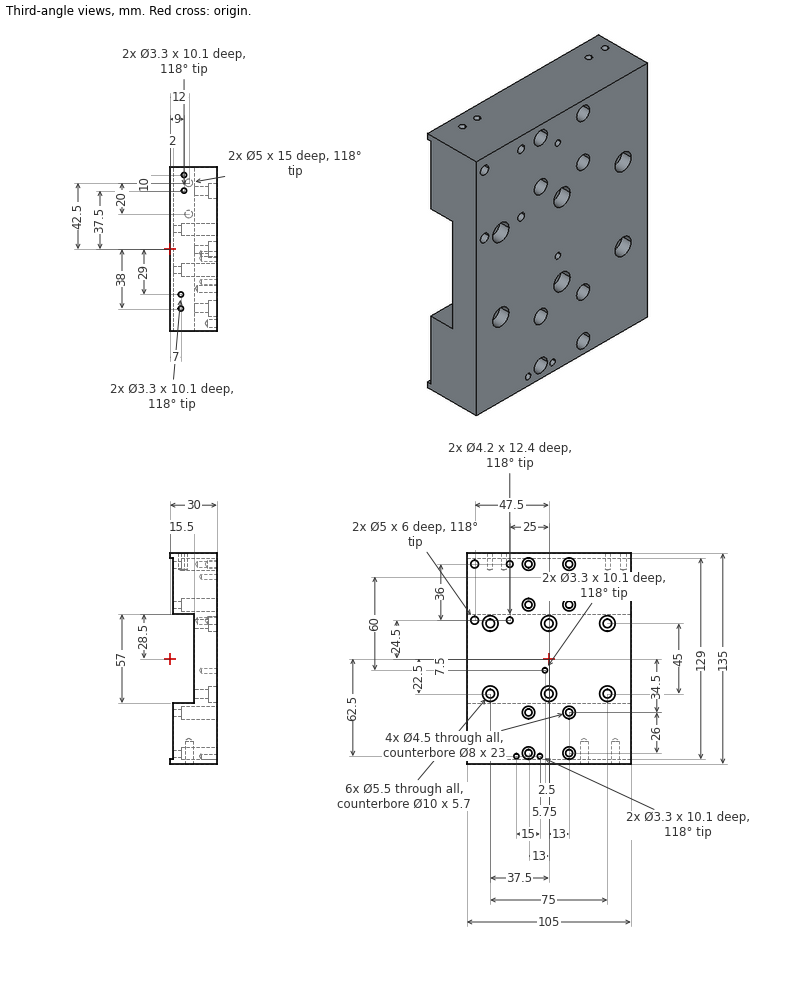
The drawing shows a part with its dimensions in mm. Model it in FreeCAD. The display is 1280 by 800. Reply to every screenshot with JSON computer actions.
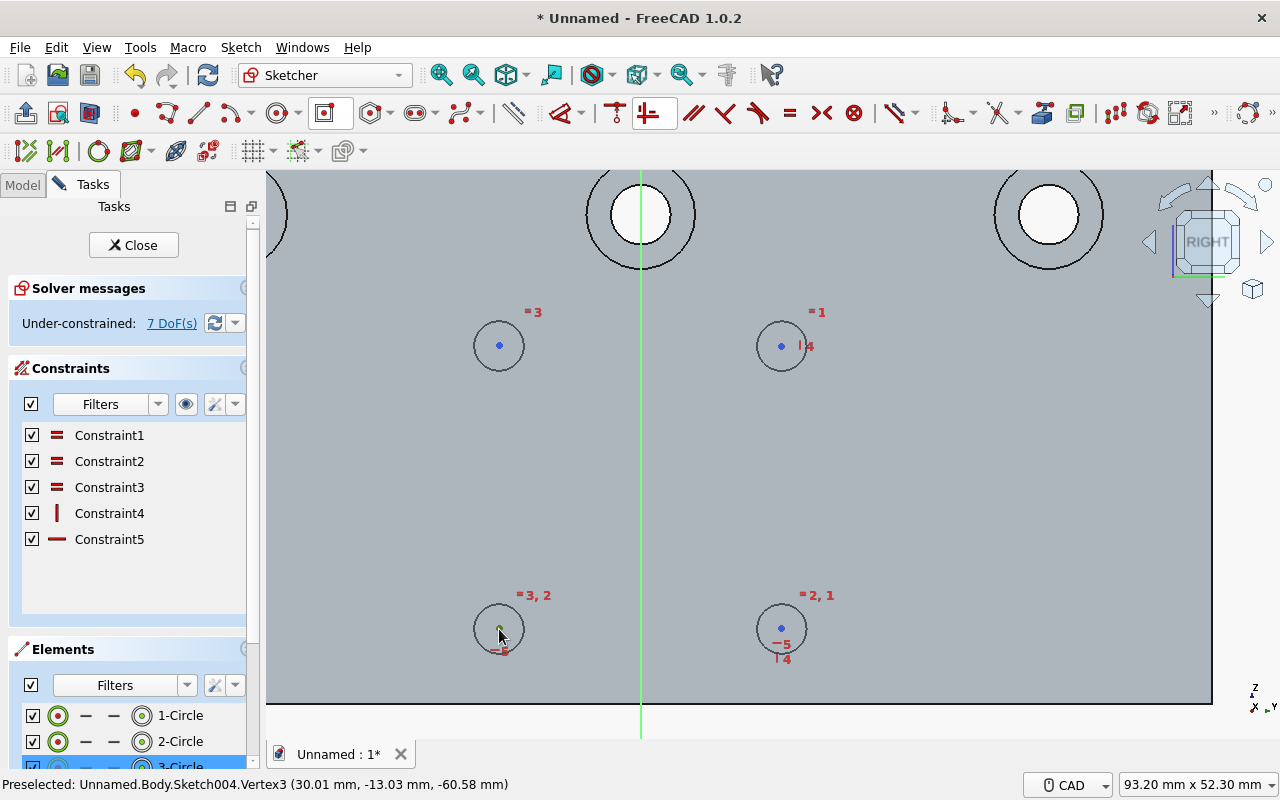
{"action": "left_click", "coordinate": [499, 346]}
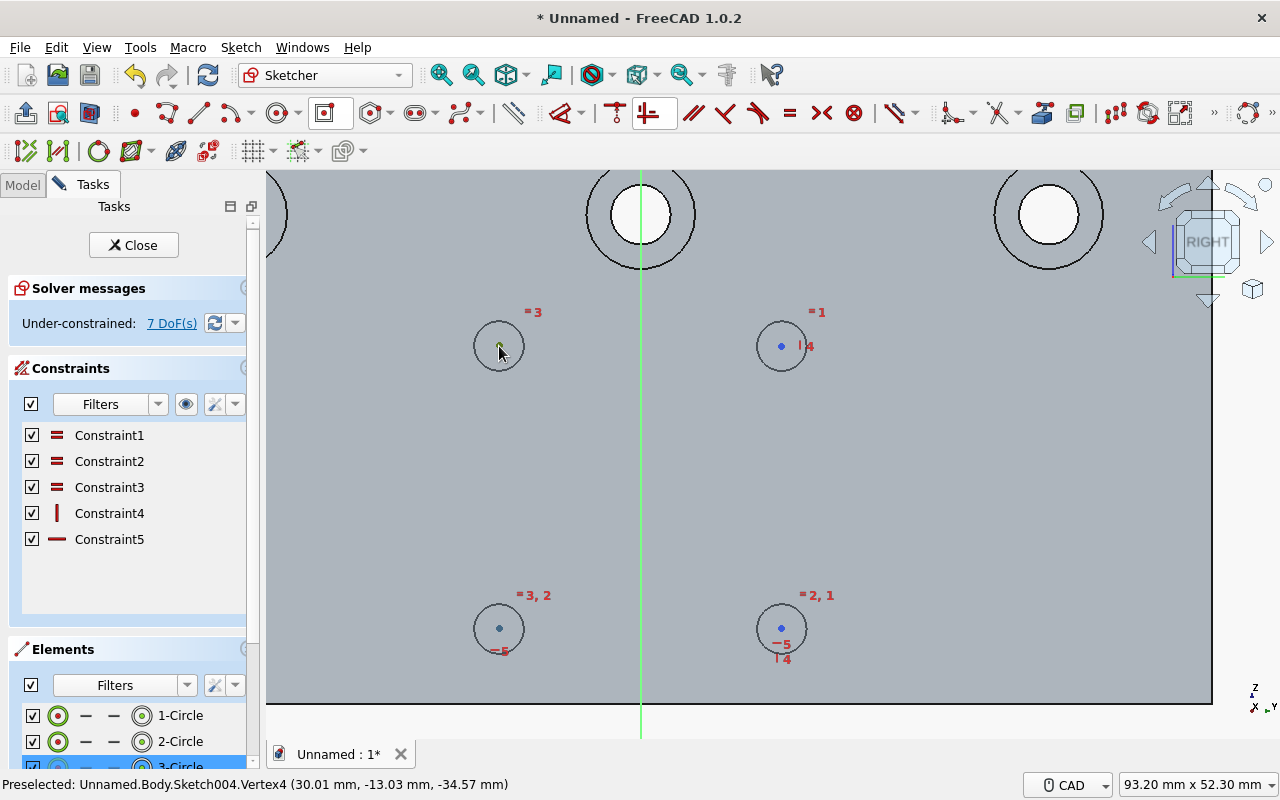
{"action": "key", "text": "v"}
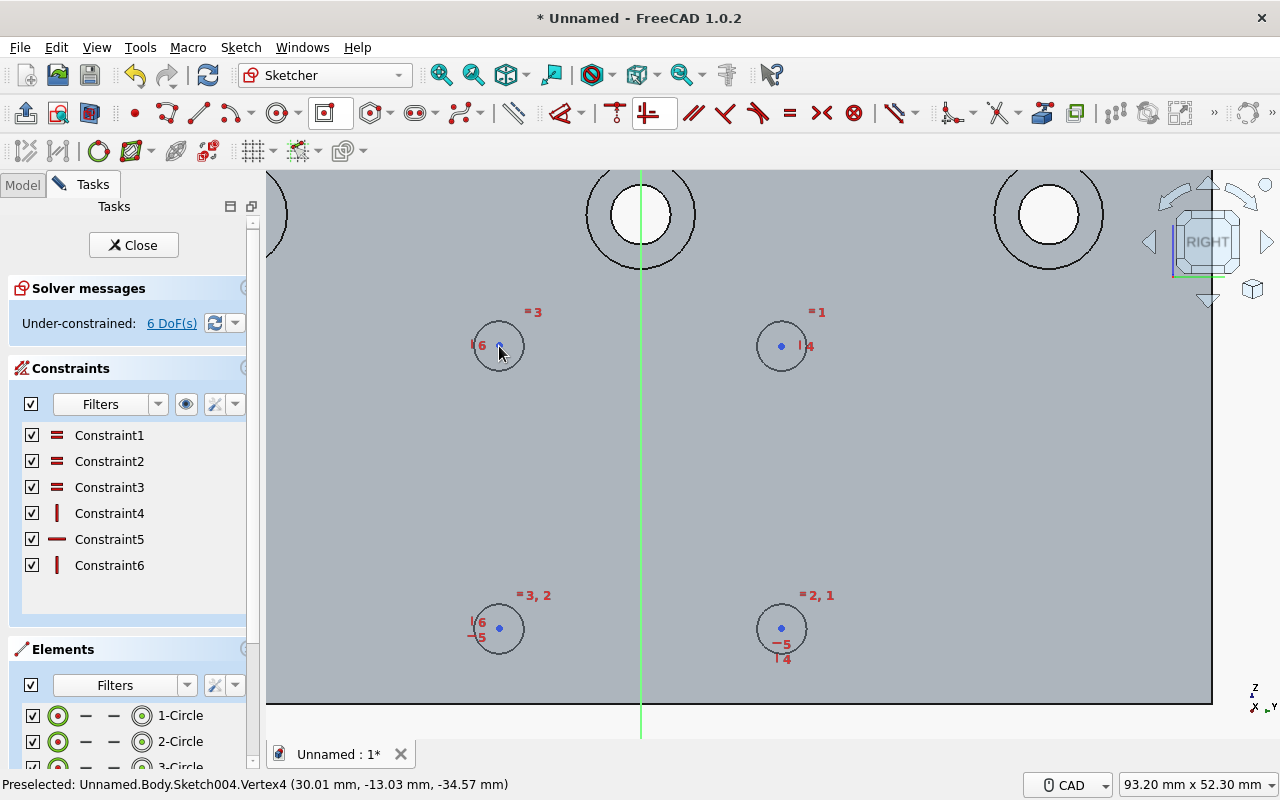
{"action": "left_click", "coordinate": [782, 346]}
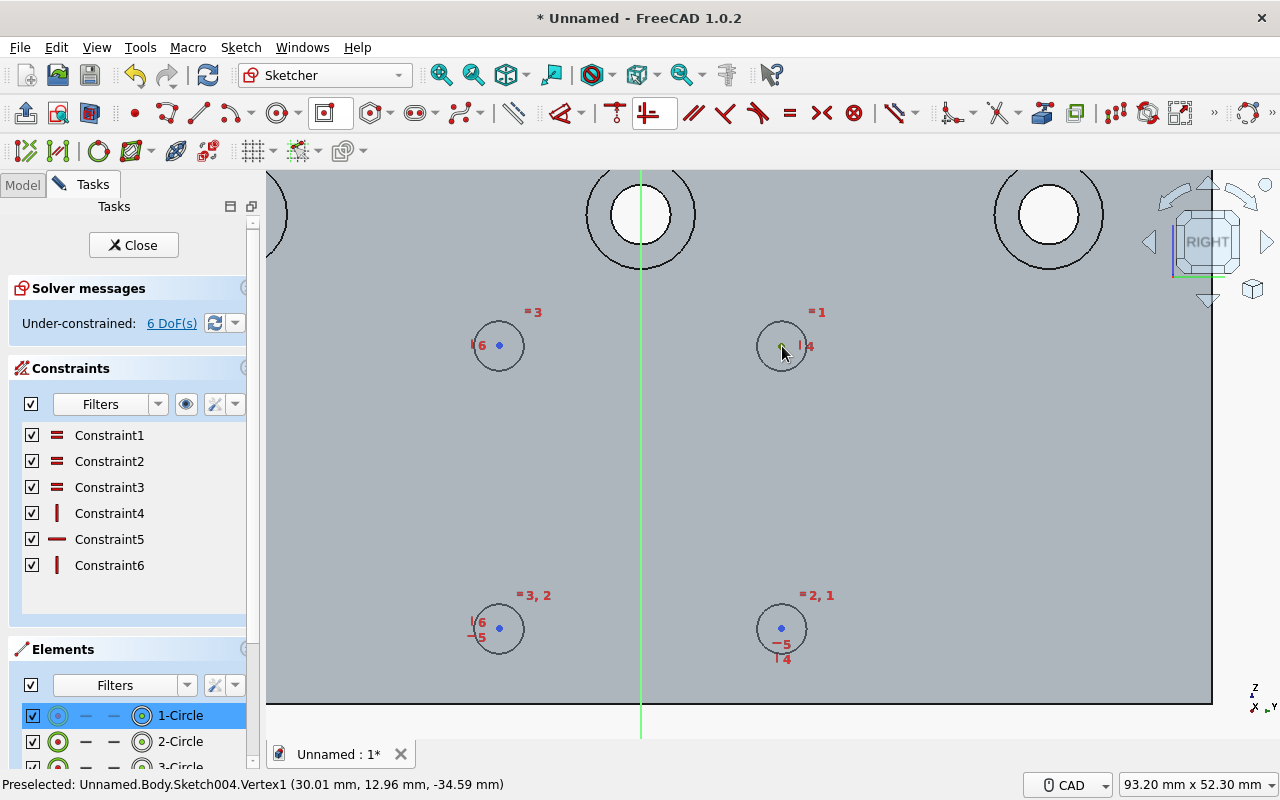
{"action": "left_click", "coordinate": [499, 346]}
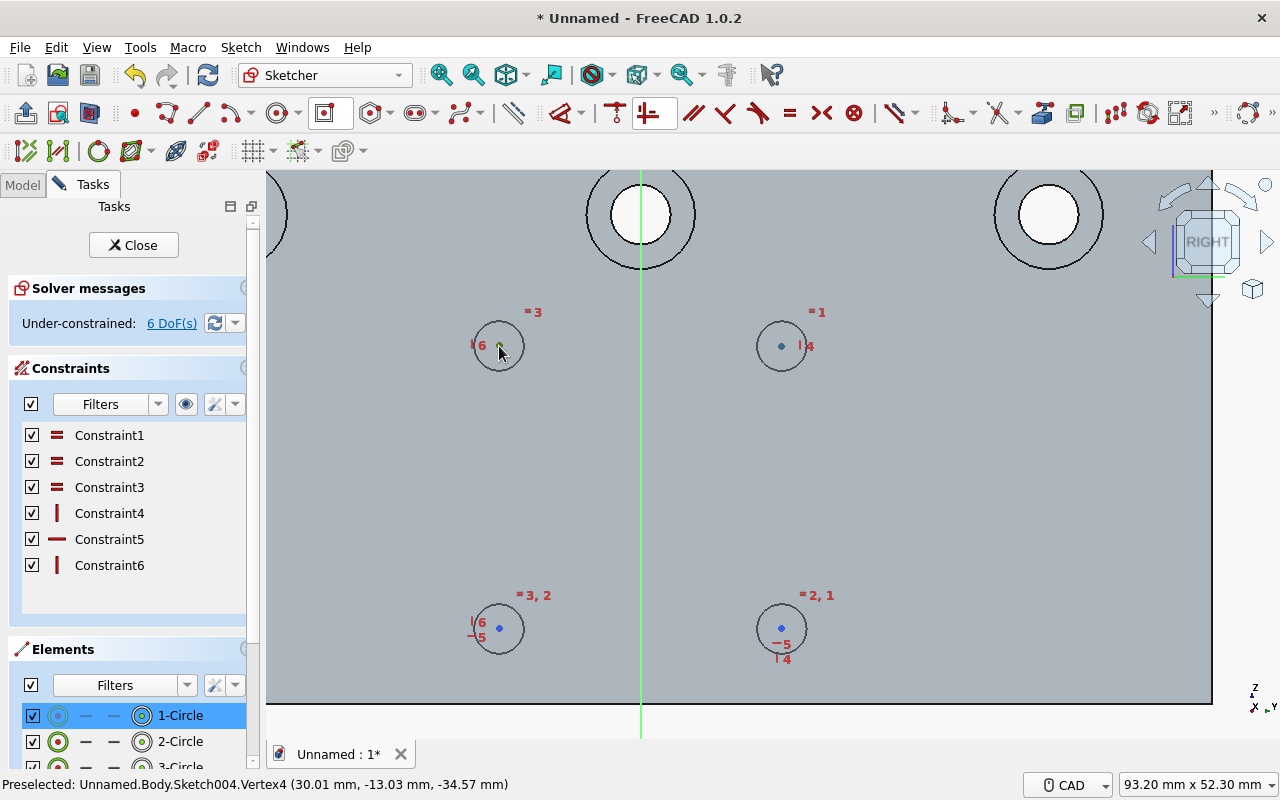
{"action": "left_click", "coordinate": [672, 114]}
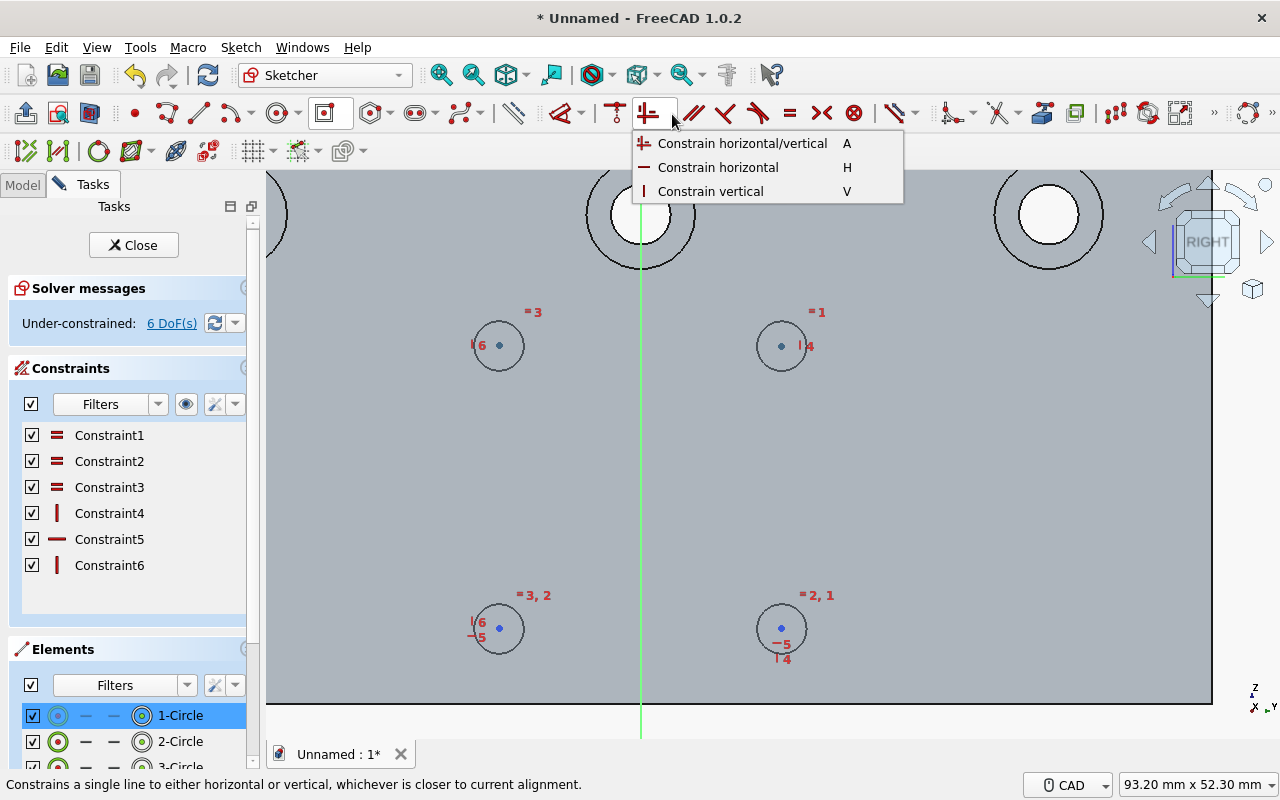
{"action": "left_click", "coordinate": [768, 167]}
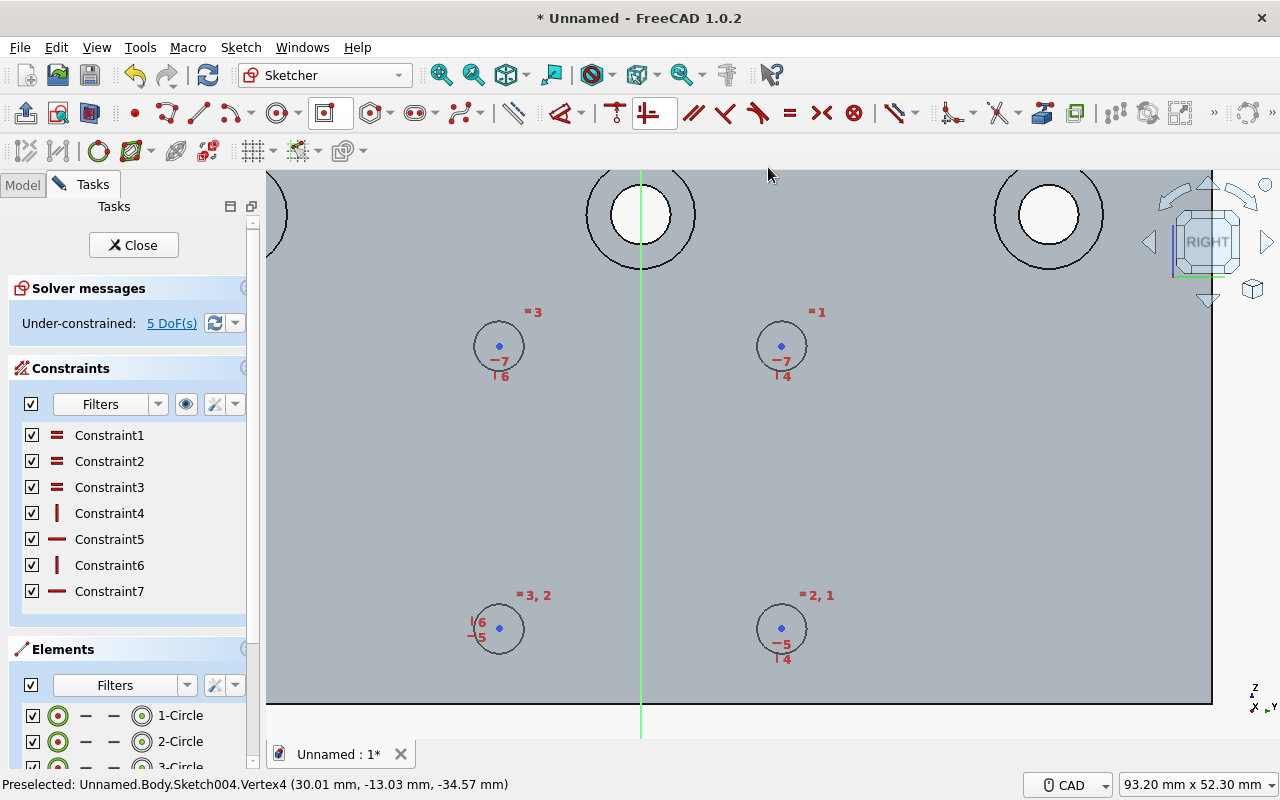
{"action": "left_click", "coordinate": [560, 114]}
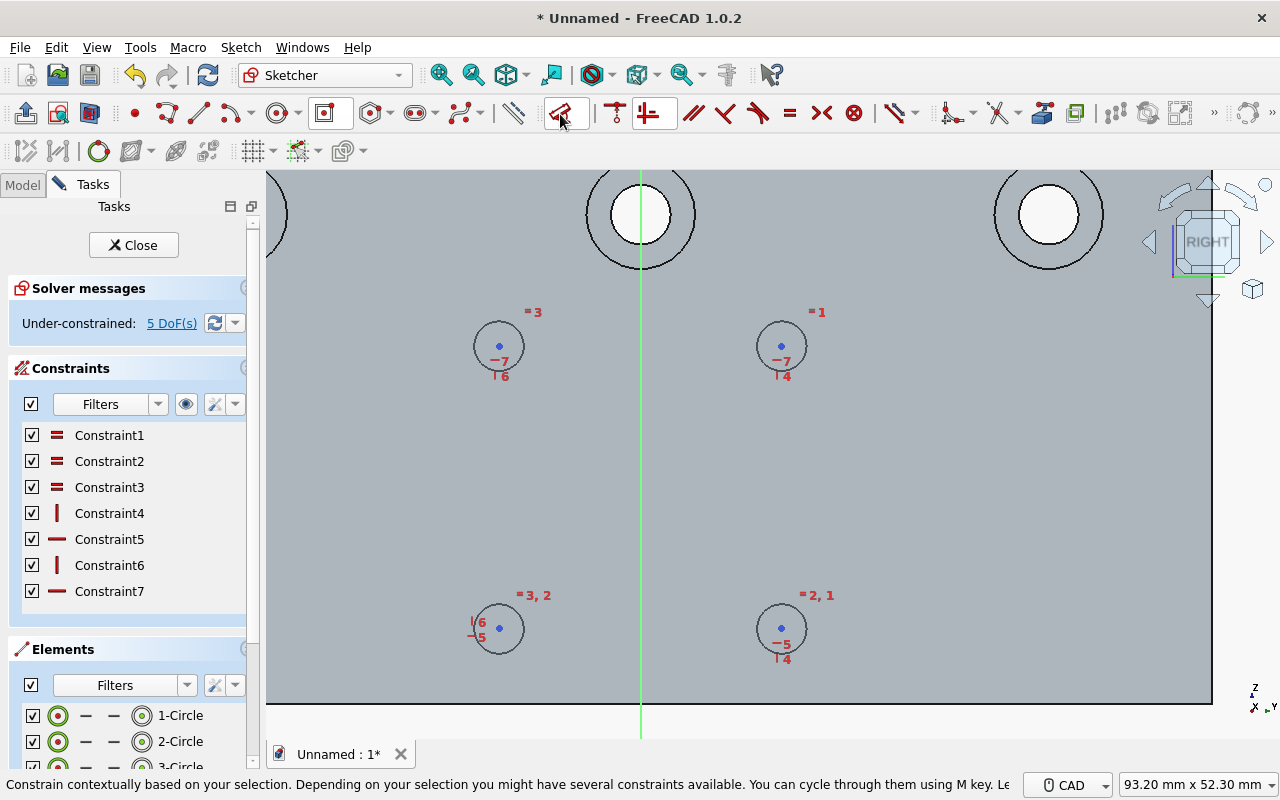
{"action": "left_click", "coordinate": [799, 329]}
{"action": "left_click", "coordinate": [822, 306]}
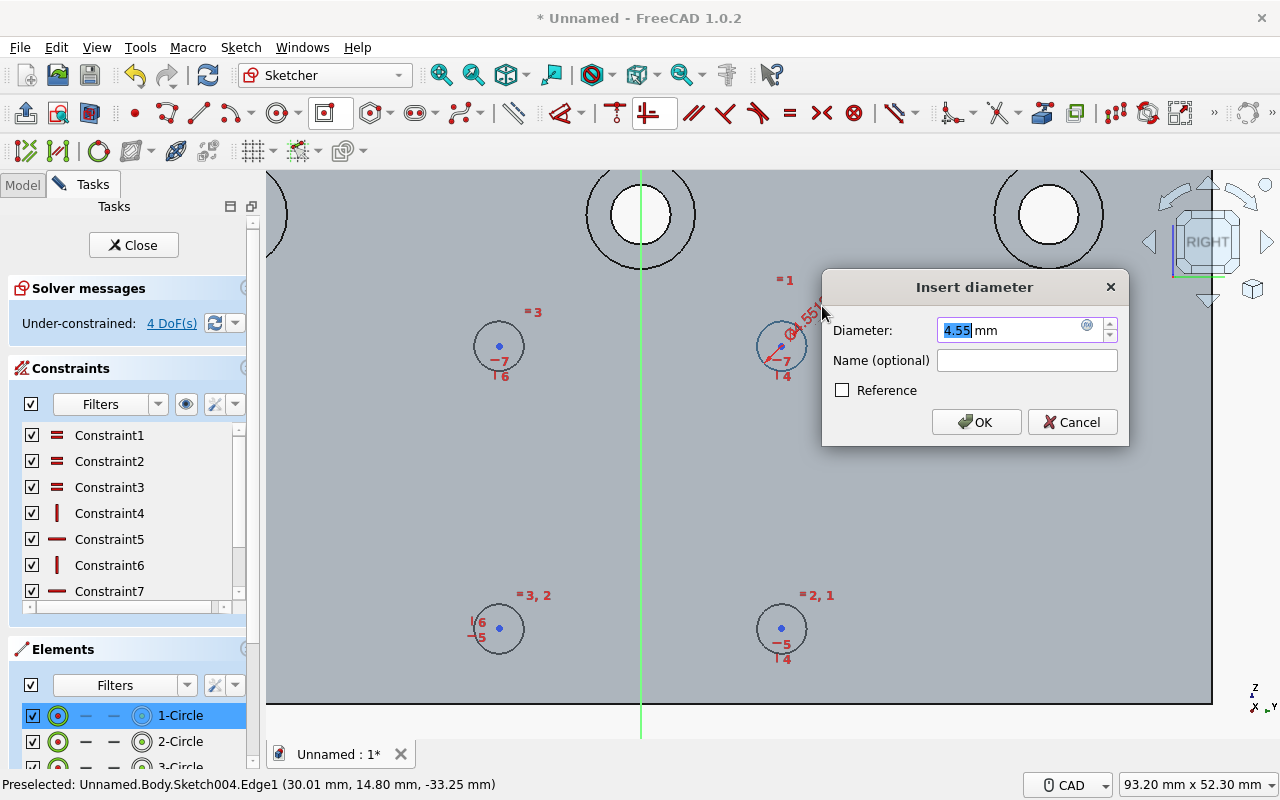
{"action": "type", "text": "4.5"}
{"action": "key", "text": "Return"}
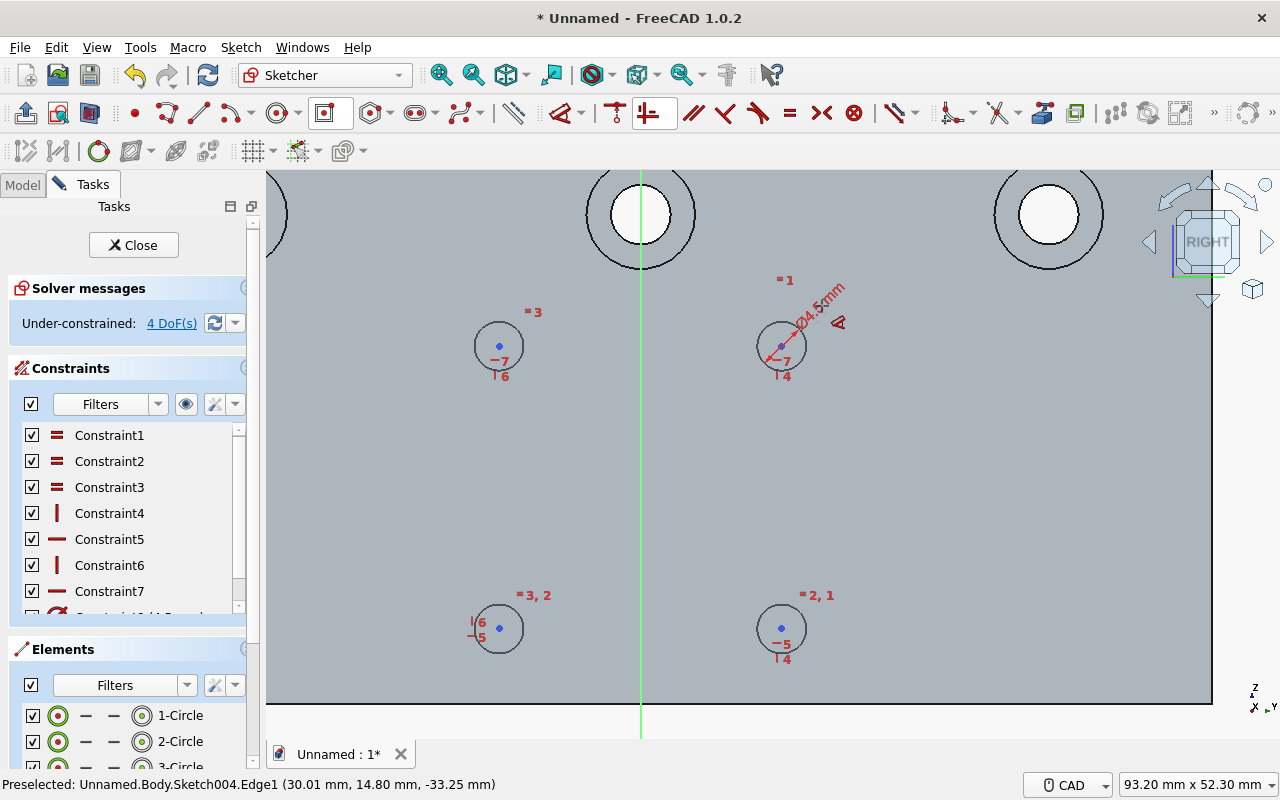
{"action": "left_click", "coordinate": [782, 346]}
{"action": "left_click", "coordinate": [711, 380]}